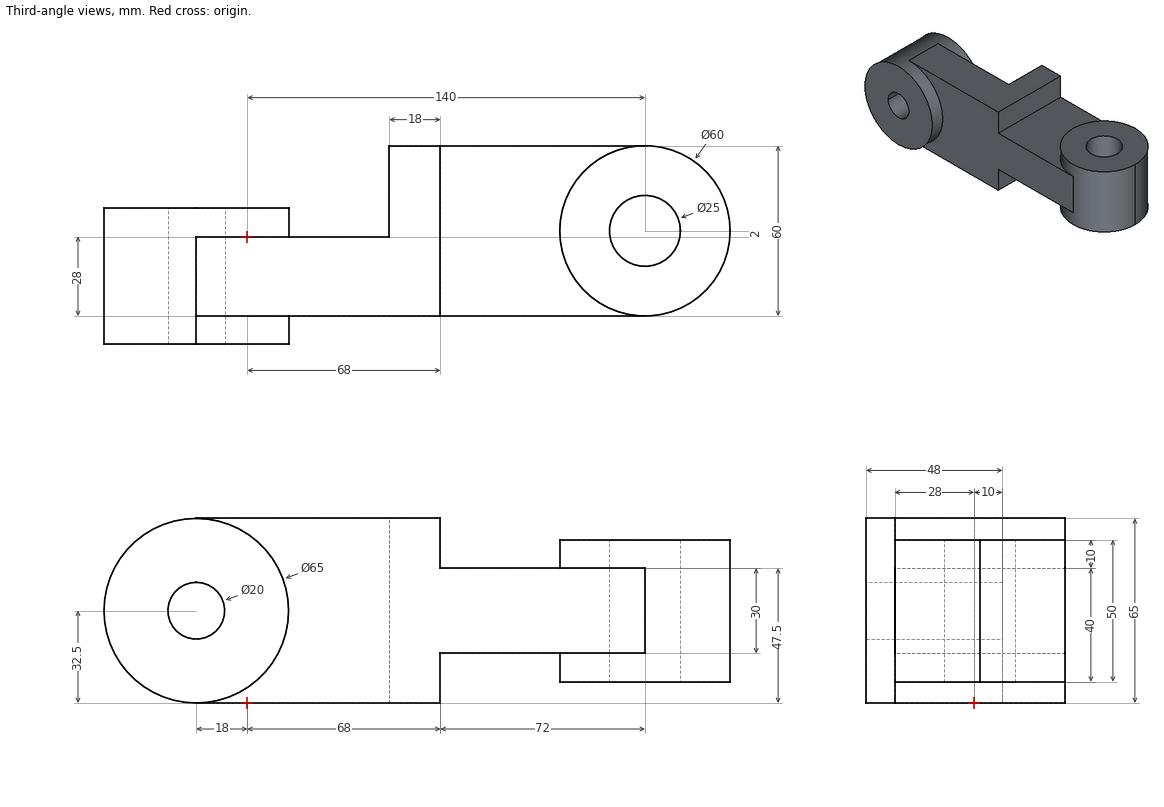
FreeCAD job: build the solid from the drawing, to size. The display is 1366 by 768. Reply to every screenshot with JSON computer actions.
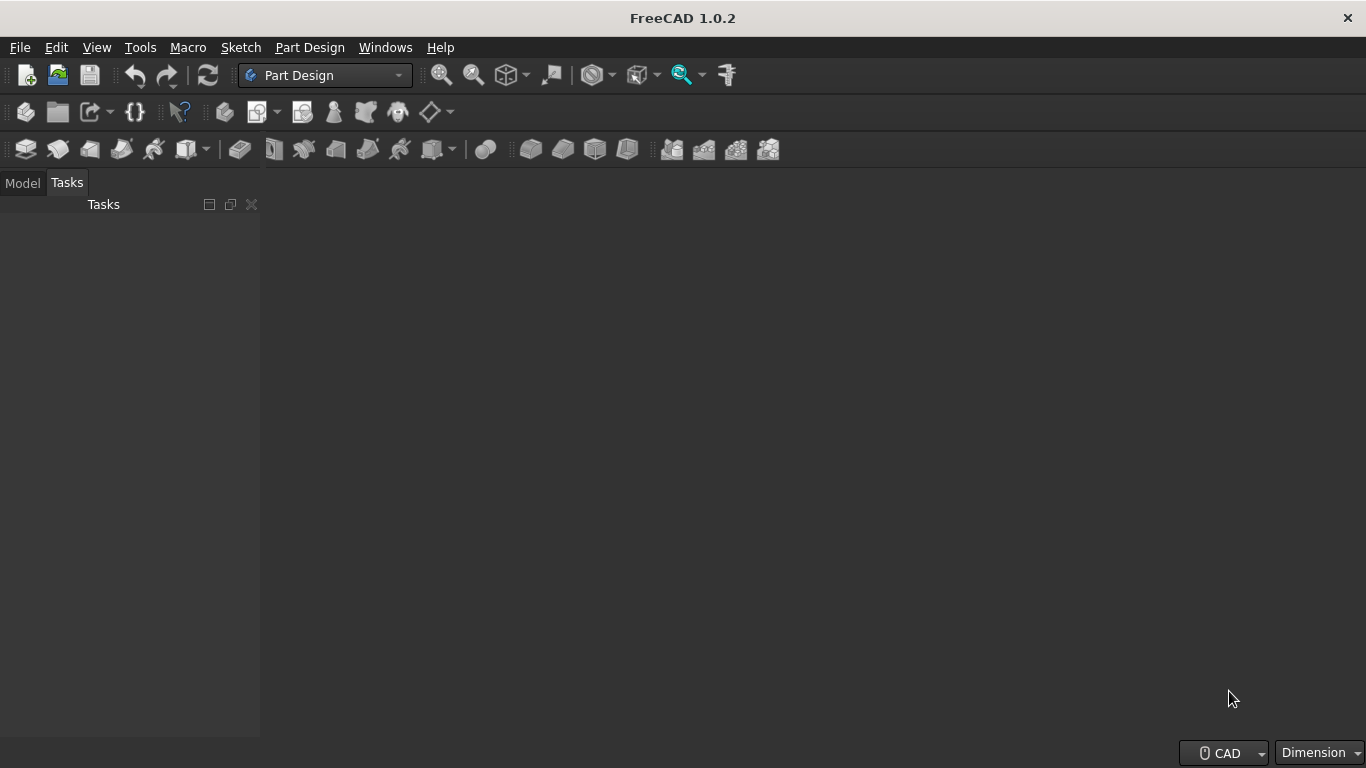
{"action": "key", "text": "ctrl+n"}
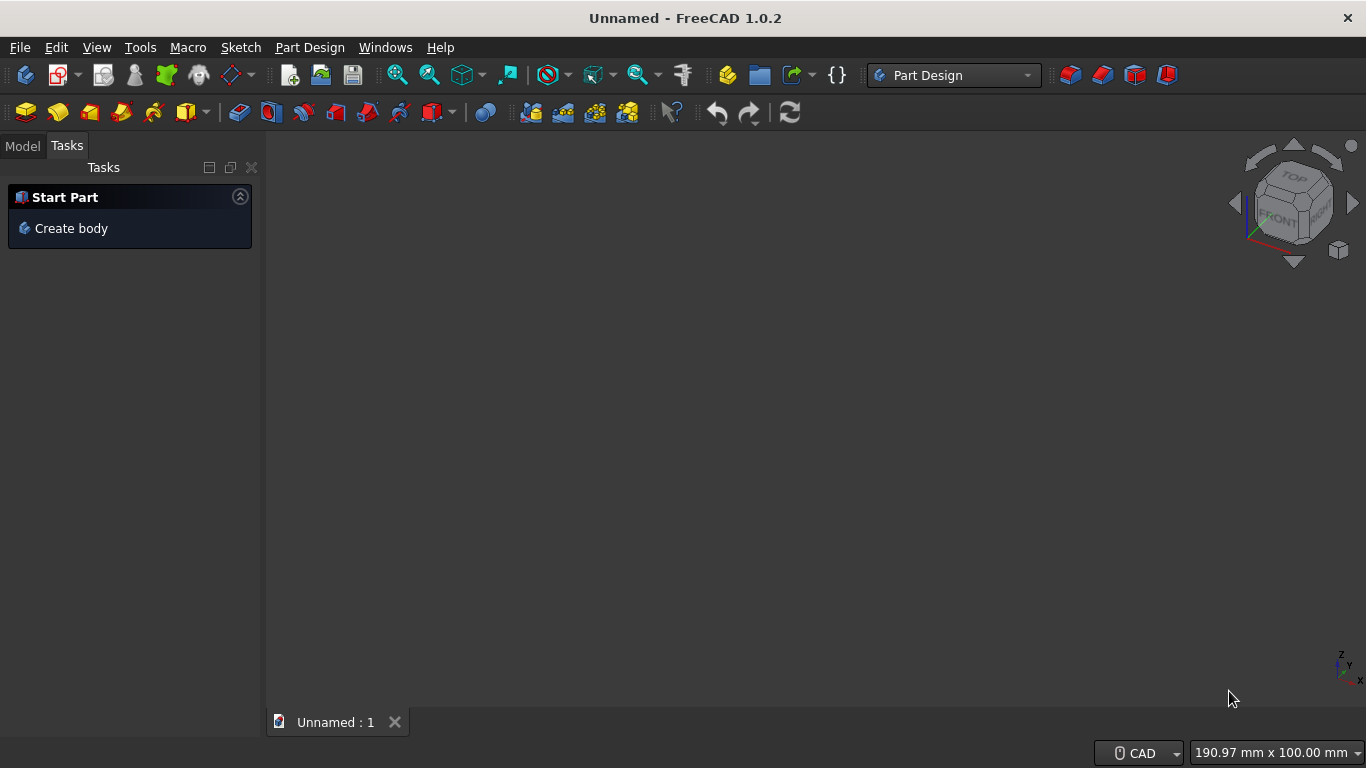
{"action": "left_click", "coordinate": [58, 76]}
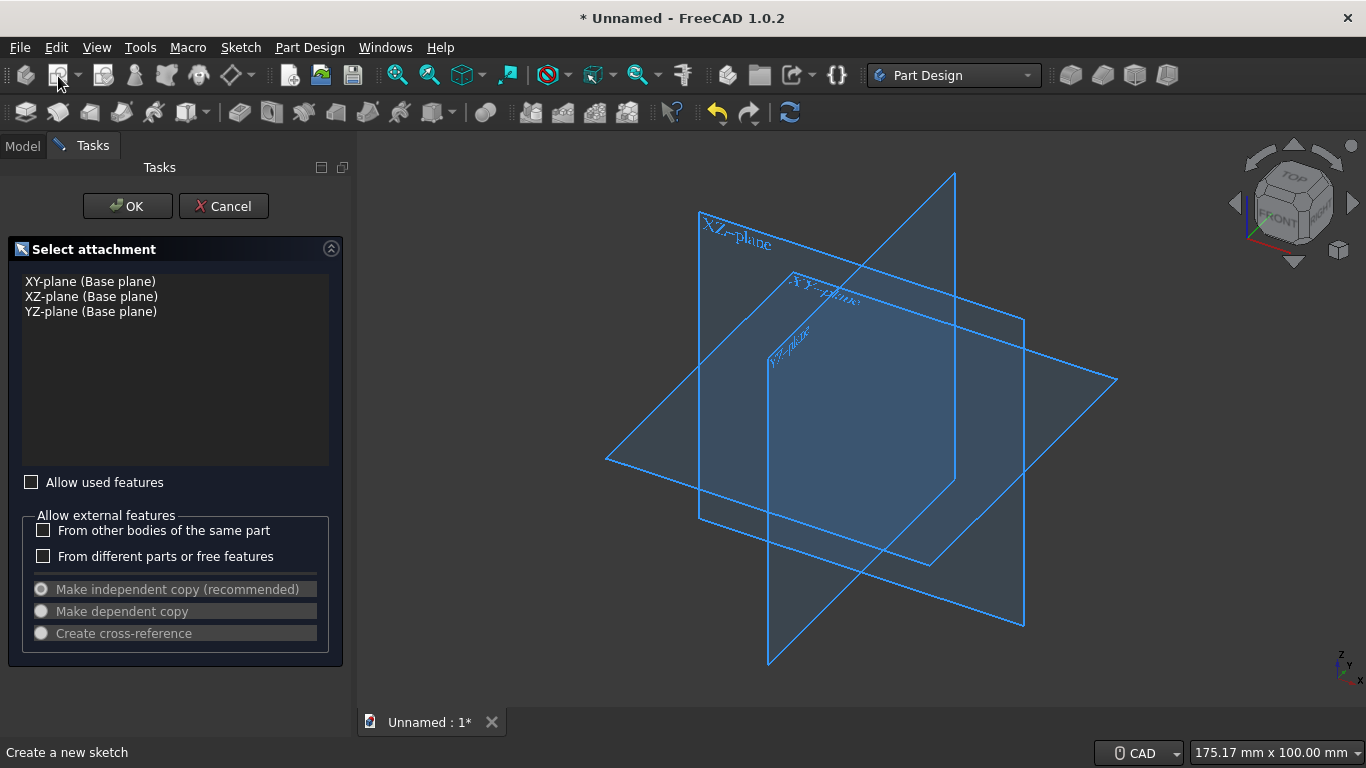
{"action": "left_click", "coordinate": [82, 282]}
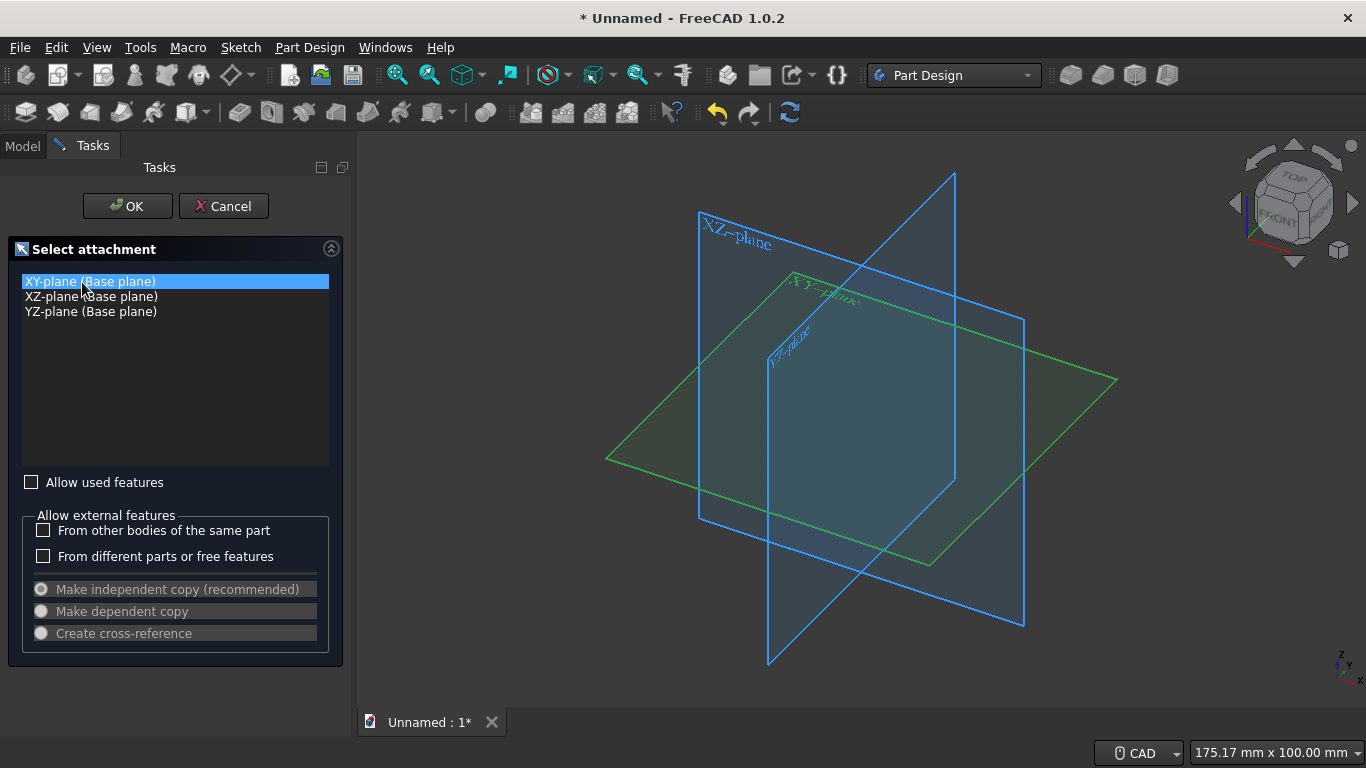
{"action": "left_click", "coordinate": [128, 206]}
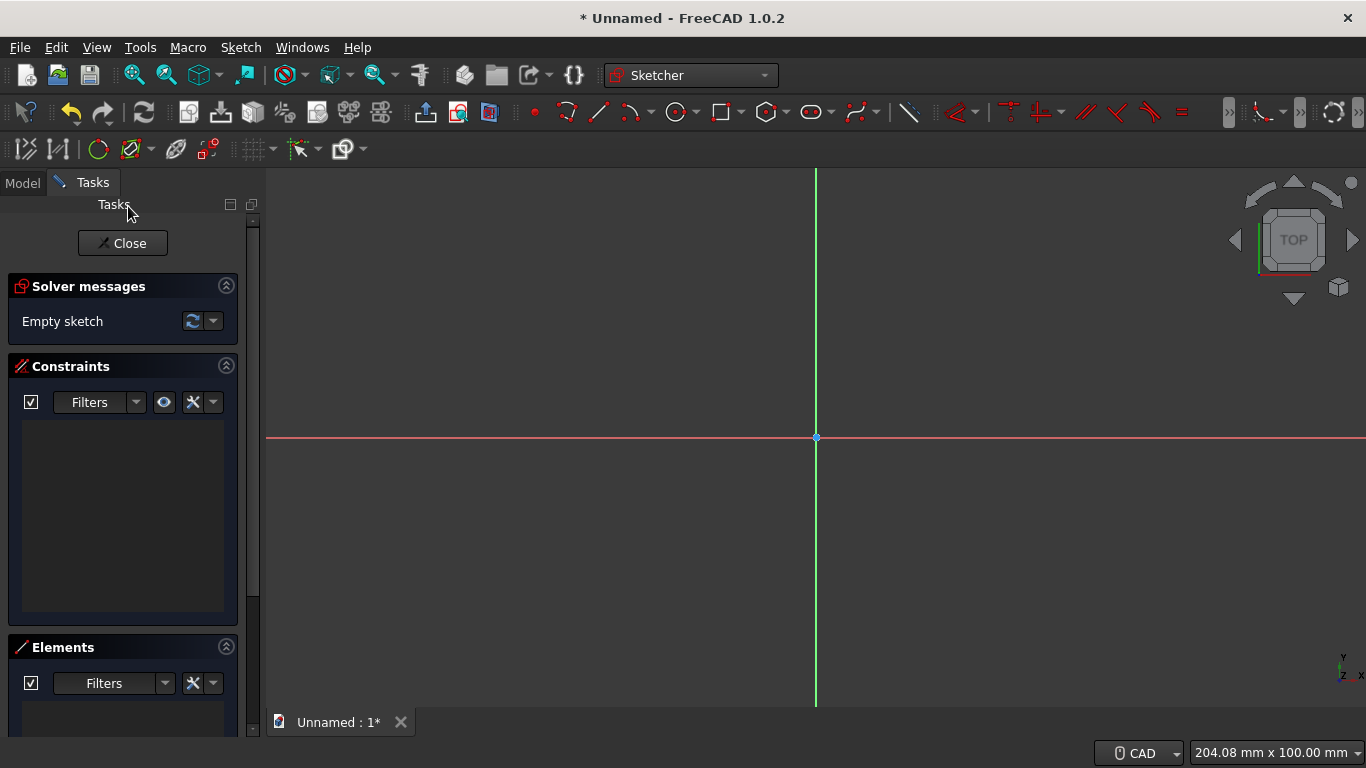
{"action": "scroll", "coordinate": [294, 486], "scroll_direction": "down", "scroll_amount": 1}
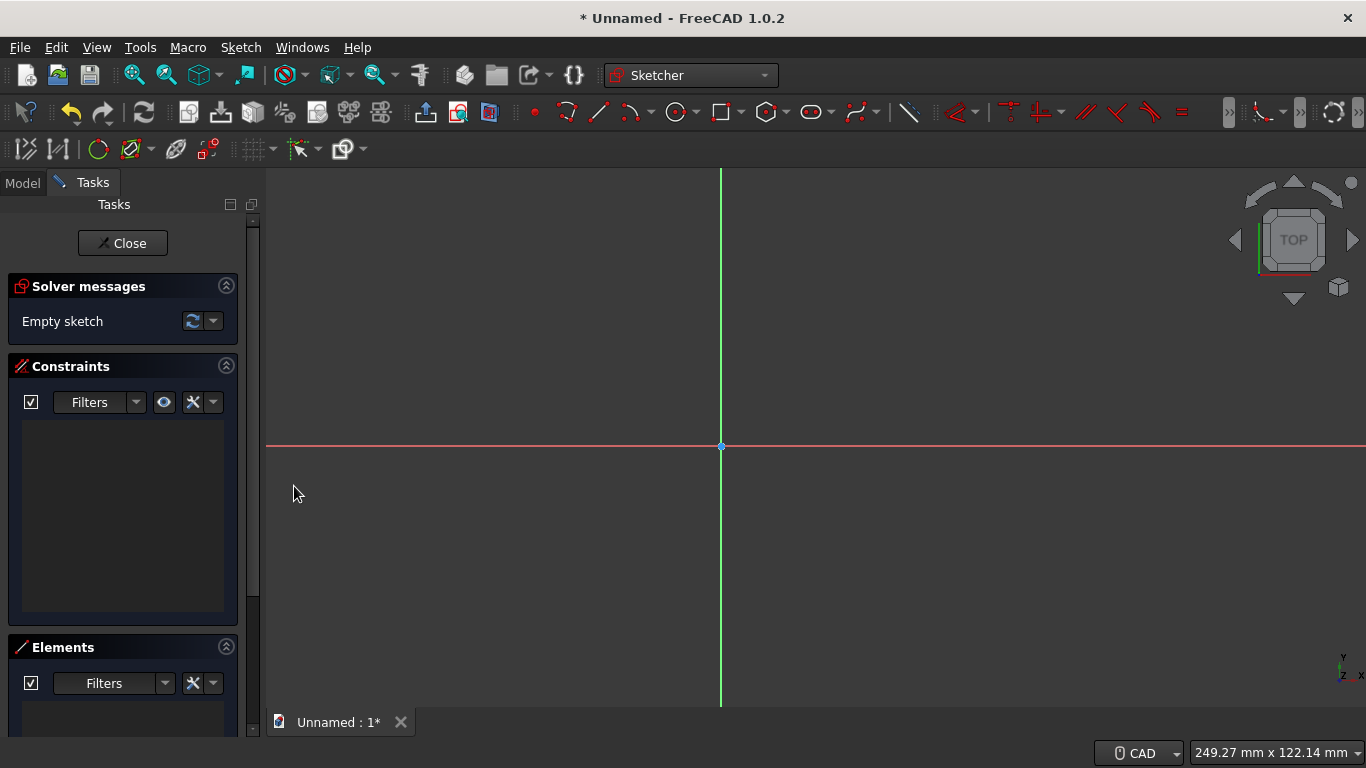
{"action": "key", "text": "g m"}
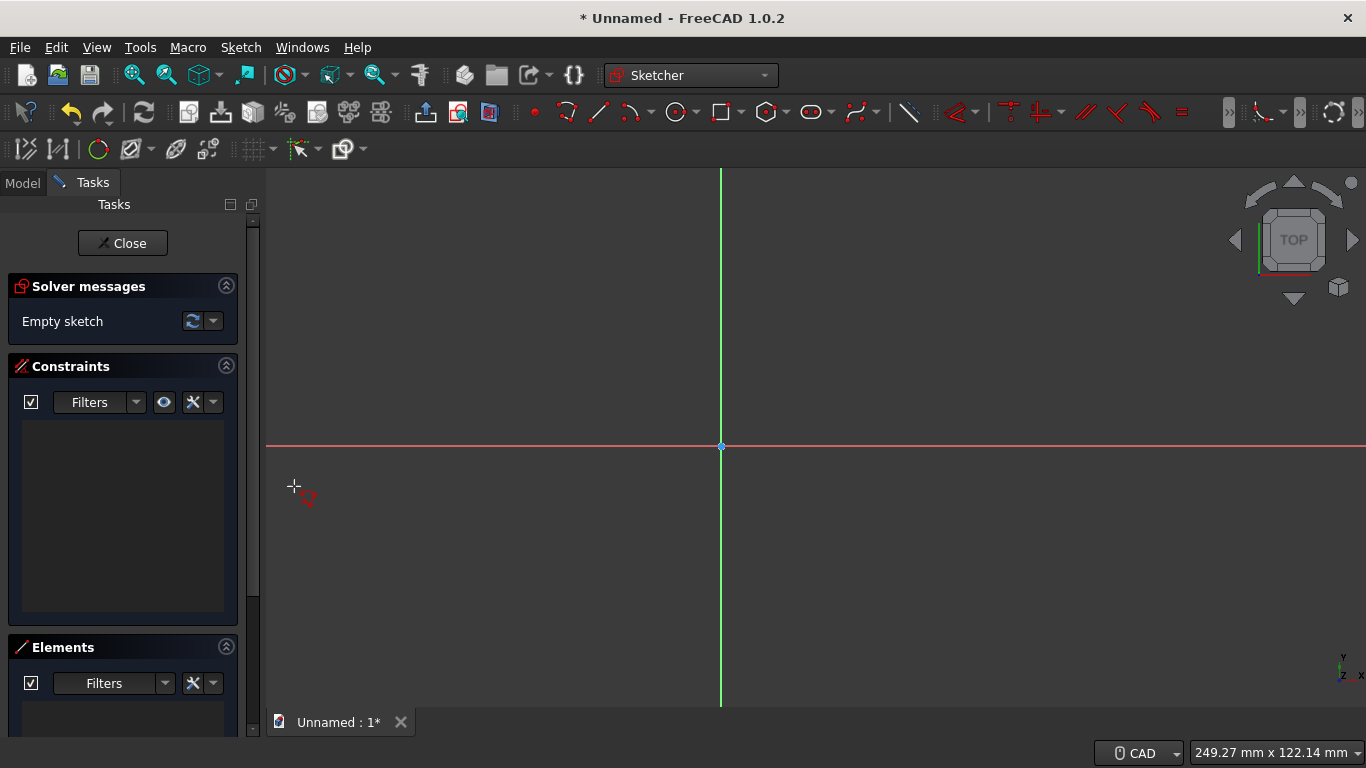
{"action": "left_click", "coordinate": [721, 446]}
{"action": "left_click", "coordinate": [730, 570]}
{"action": "left_click", "coordinate": [1021, 570]}
{"action": "left_click", "coordinate": [1021, 305]}
{"action": "left_click", "coordinate": [942, 305]}
{"action": "left_click", "coordinate": [942, 437]}
{"action": "left_click", "coordinate": [721, 446]}
{"action": "key", "text": "Escape"}
{"action": "key", "text": "Escape"}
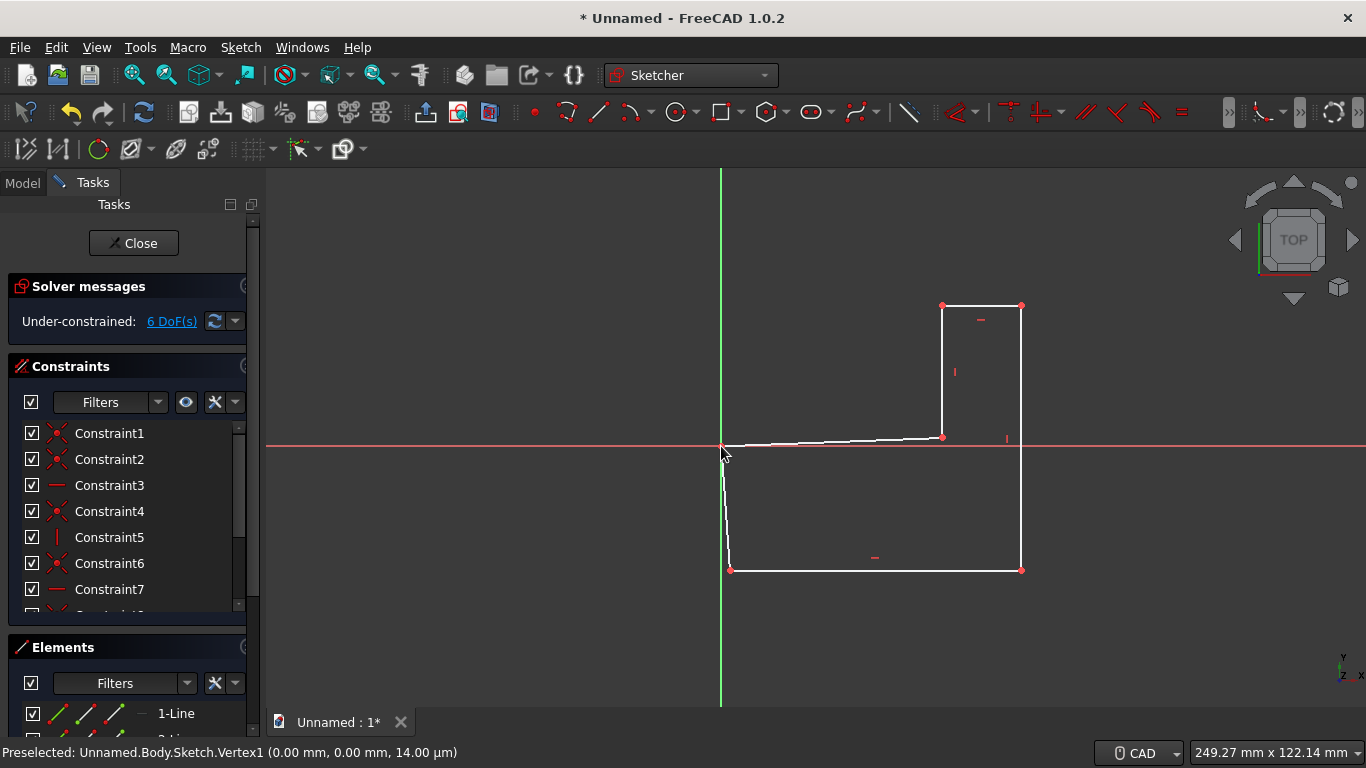
{"action": "left_click", "coordinate": [724, 484]}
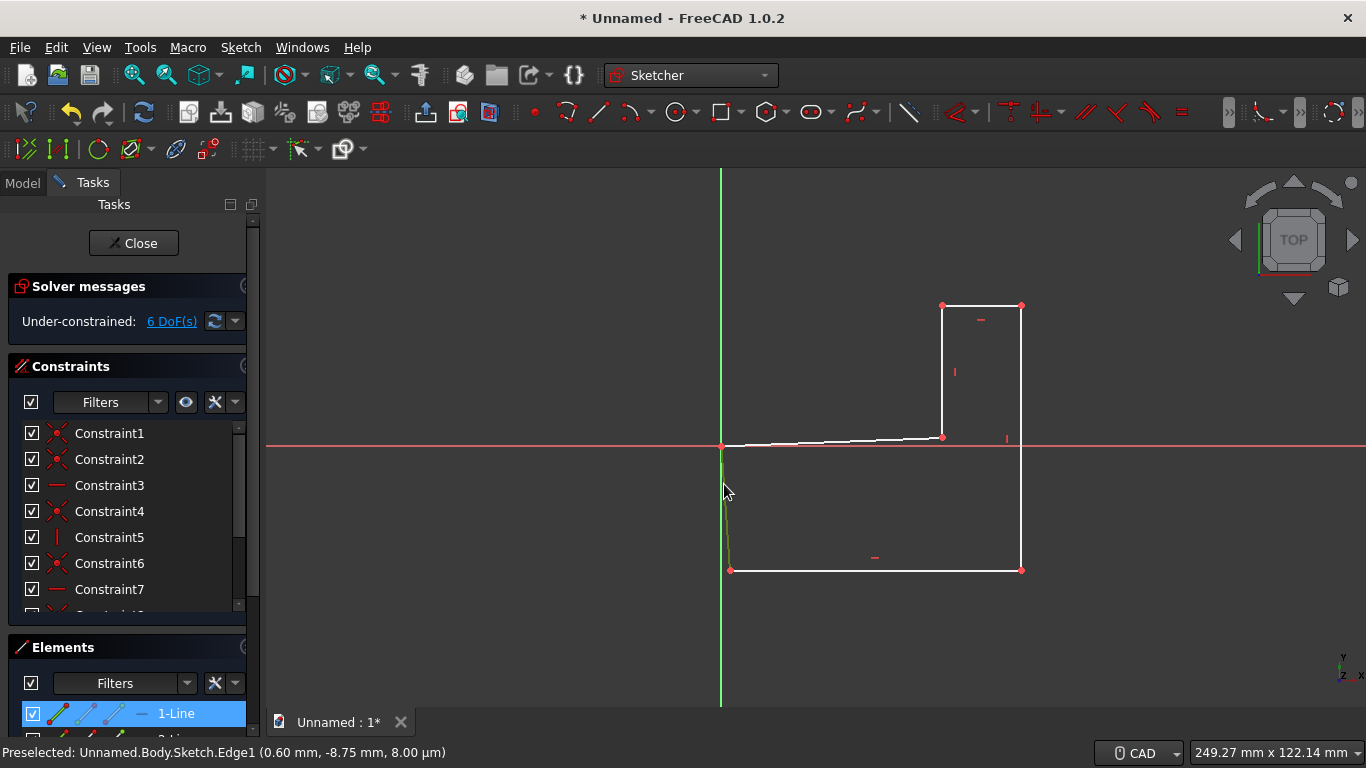
{"action": "key", "text": "v"}